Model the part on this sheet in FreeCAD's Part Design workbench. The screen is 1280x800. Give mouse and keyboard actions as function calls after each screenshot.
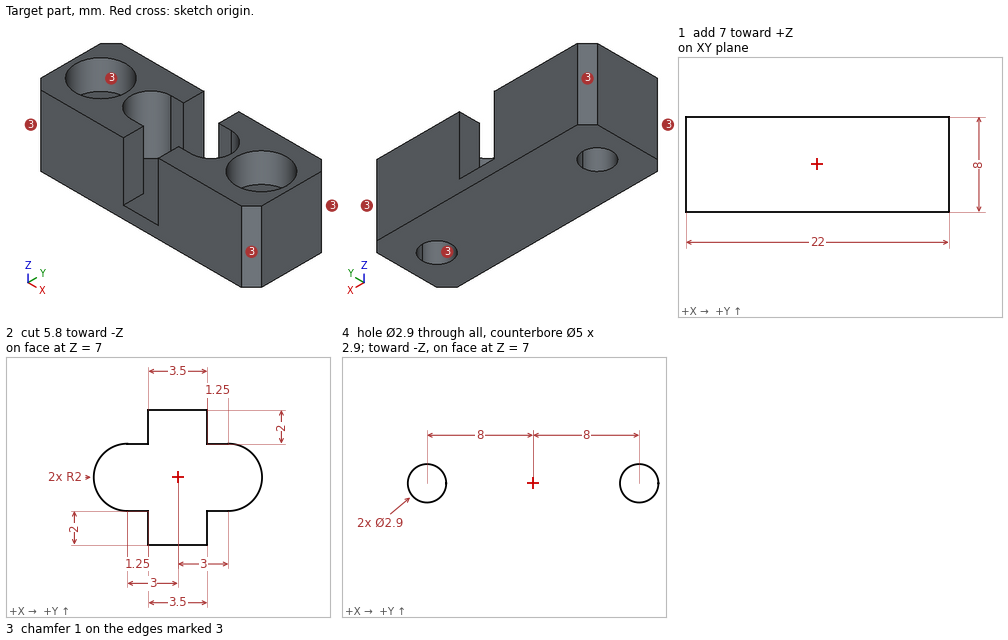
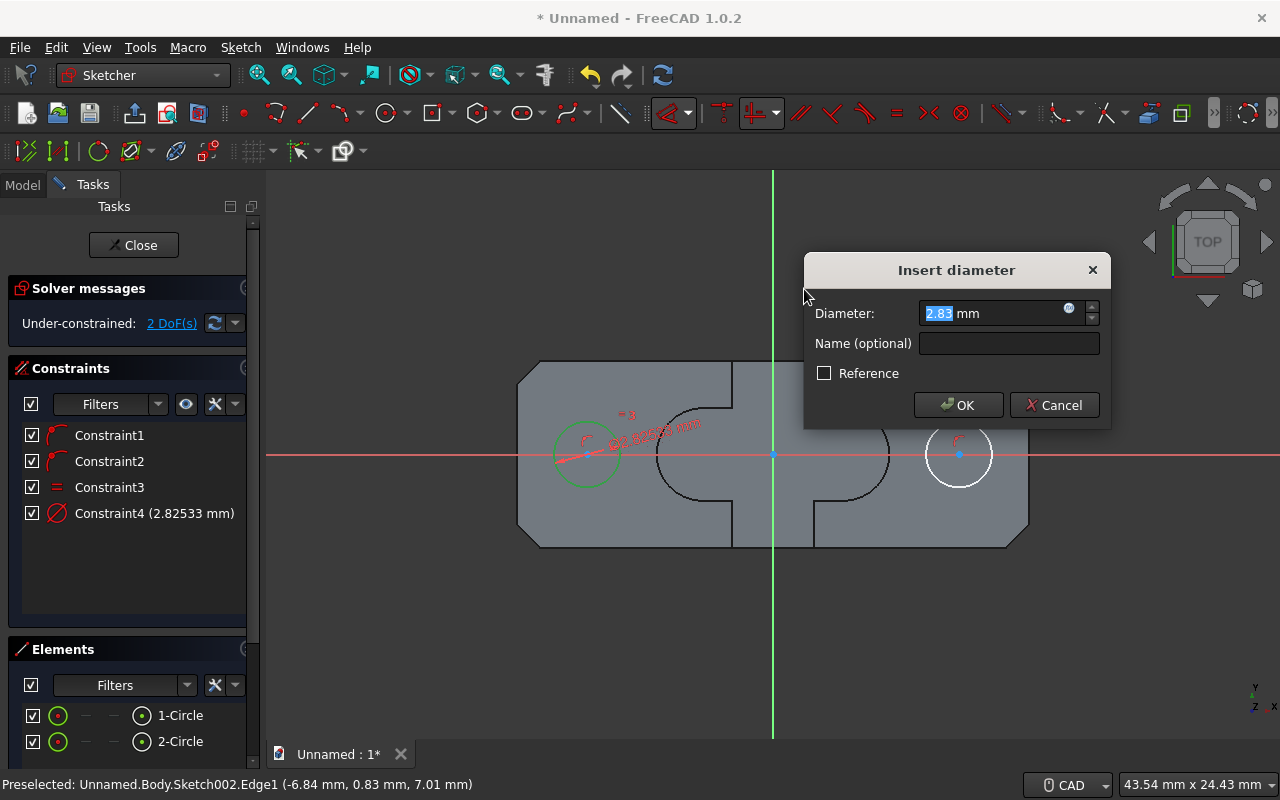
text(2.9)
key(Return)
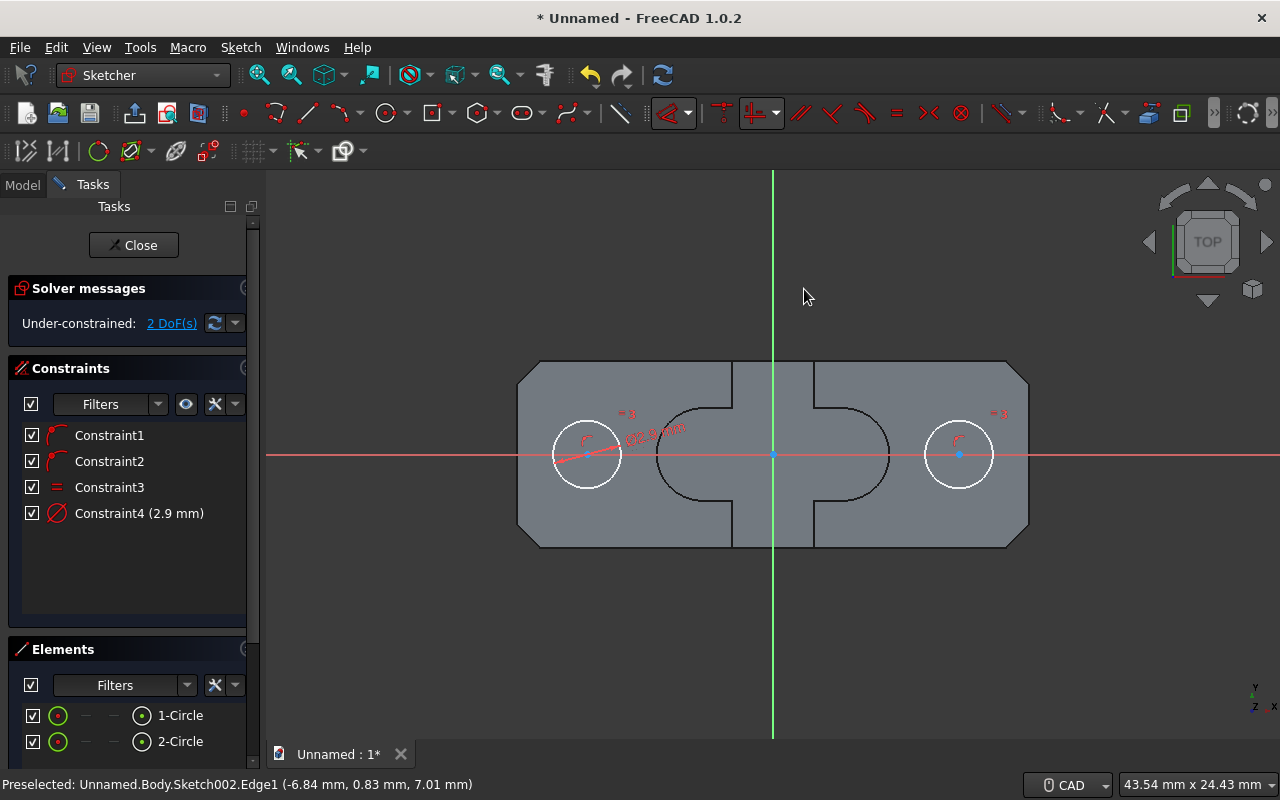
click(587, 455)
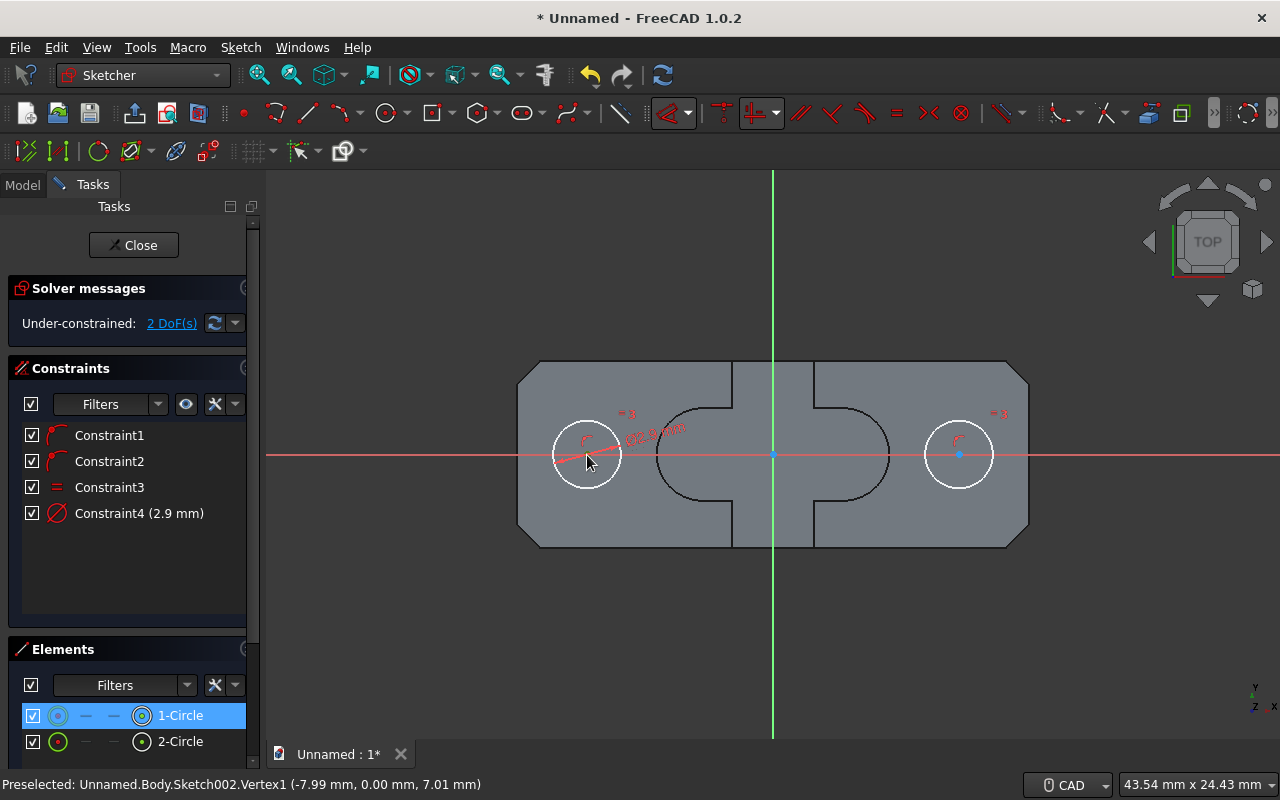
click(690, 114)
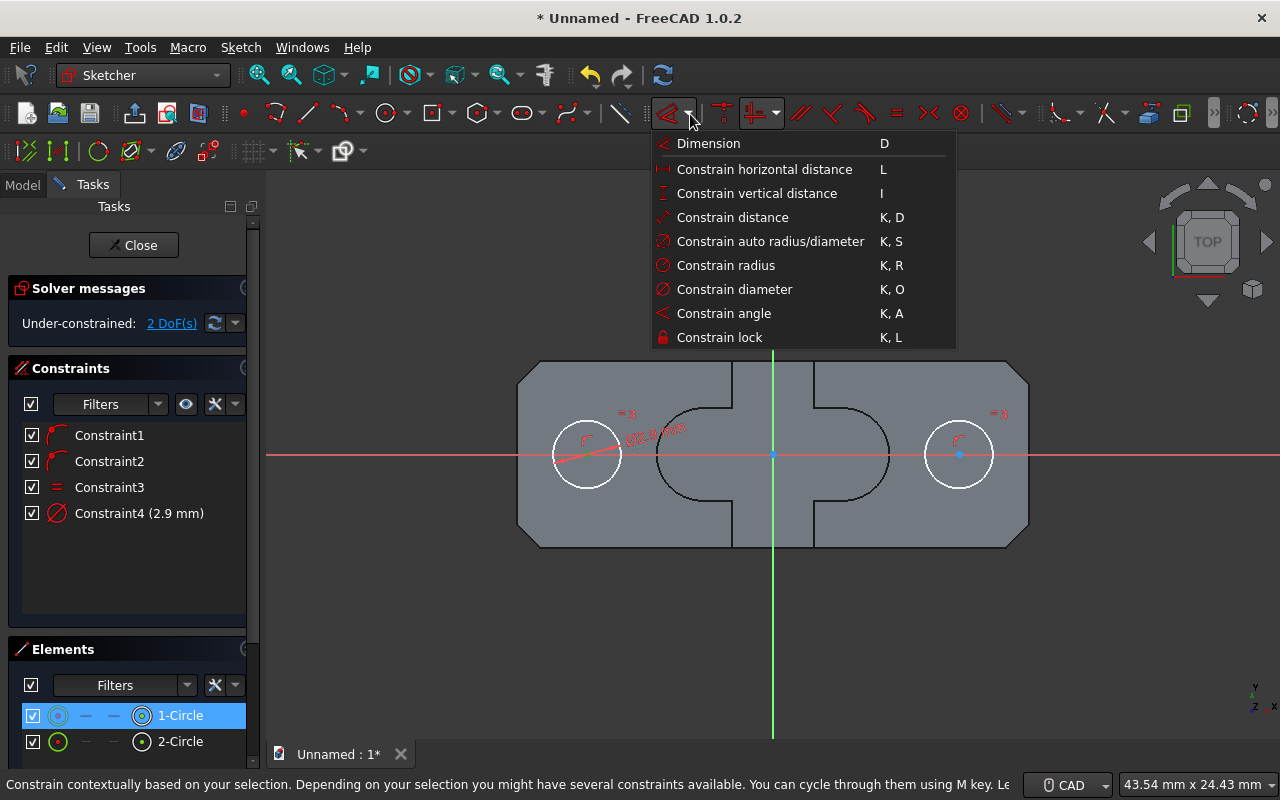
click(804, 169)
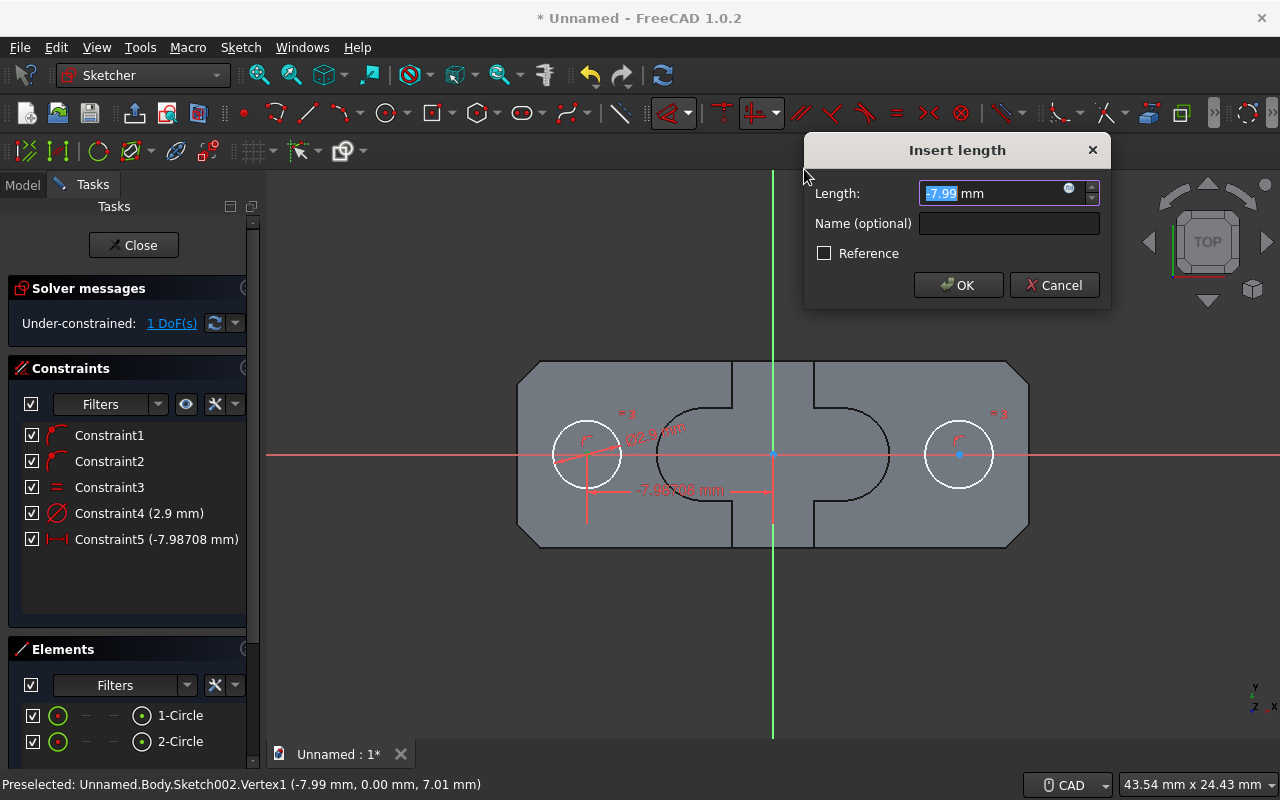
text(-8)
key(Return)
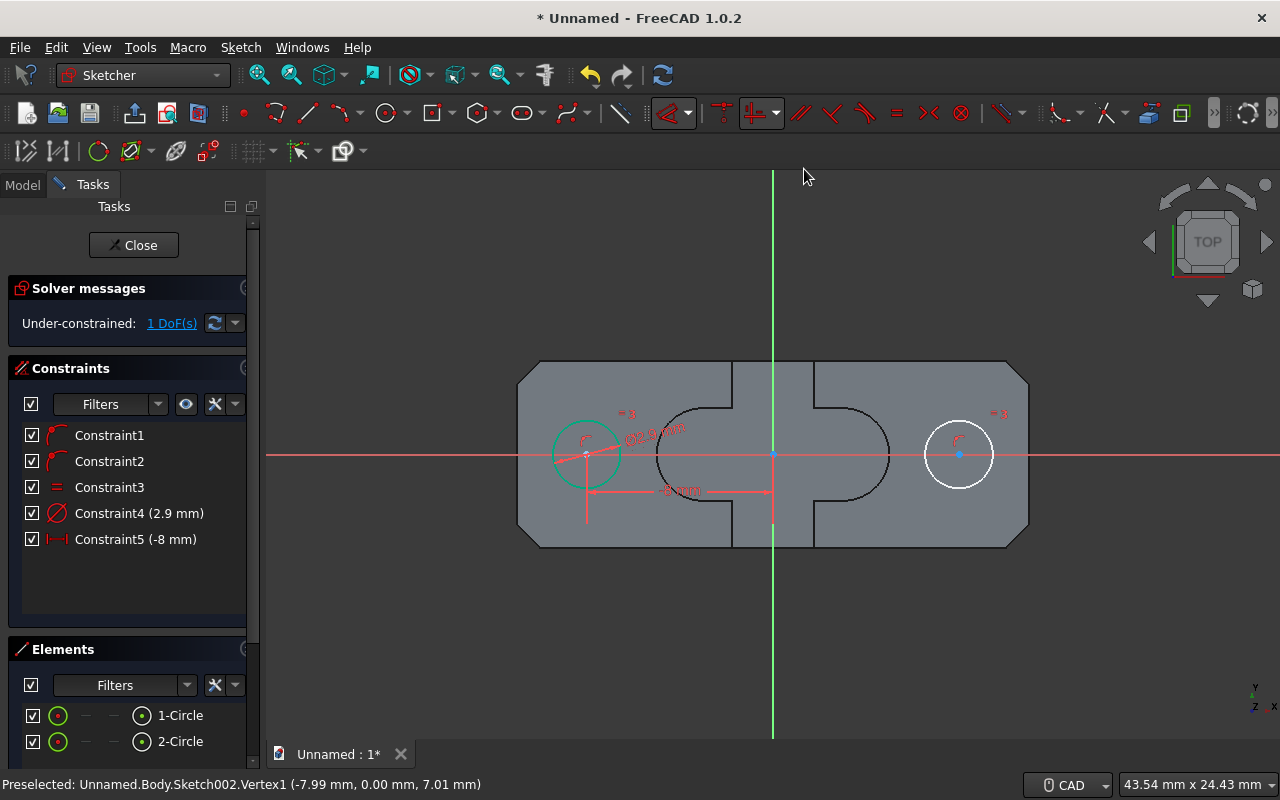
click(959, 455)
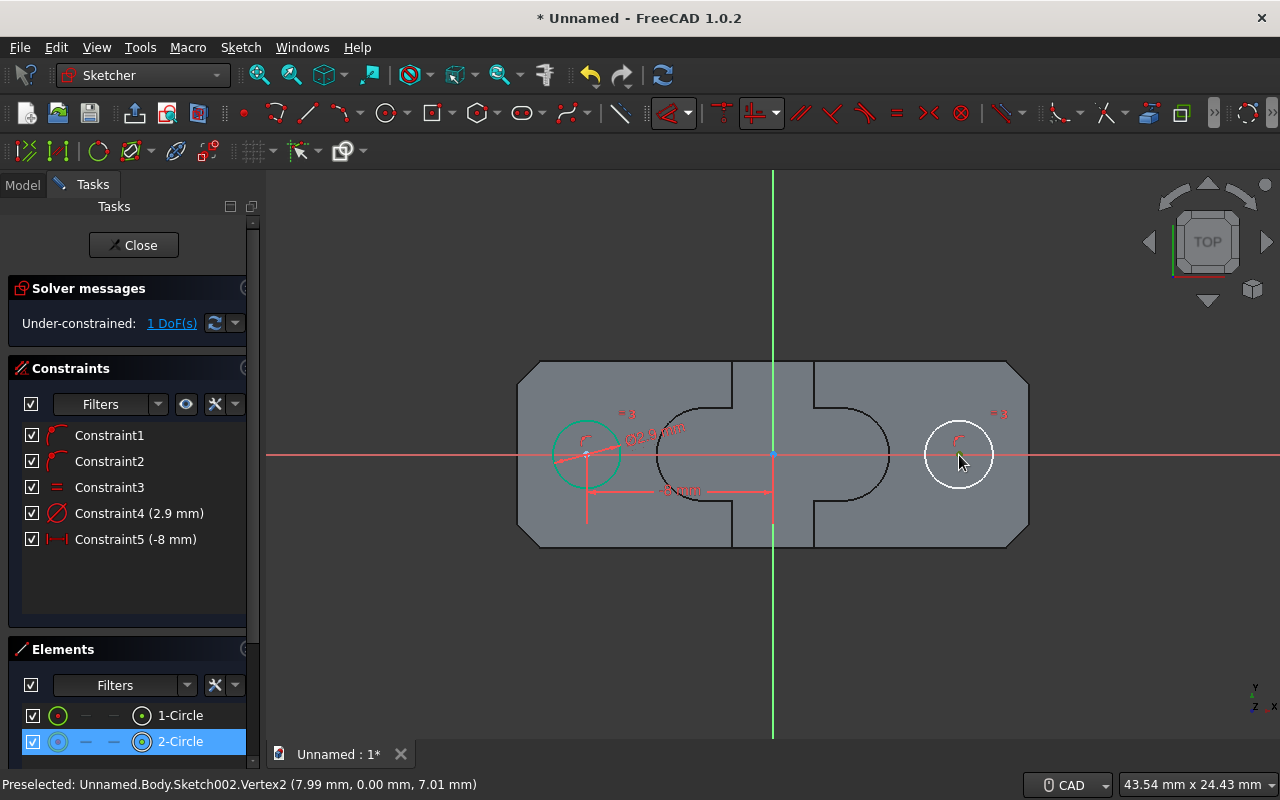
click(690, 114)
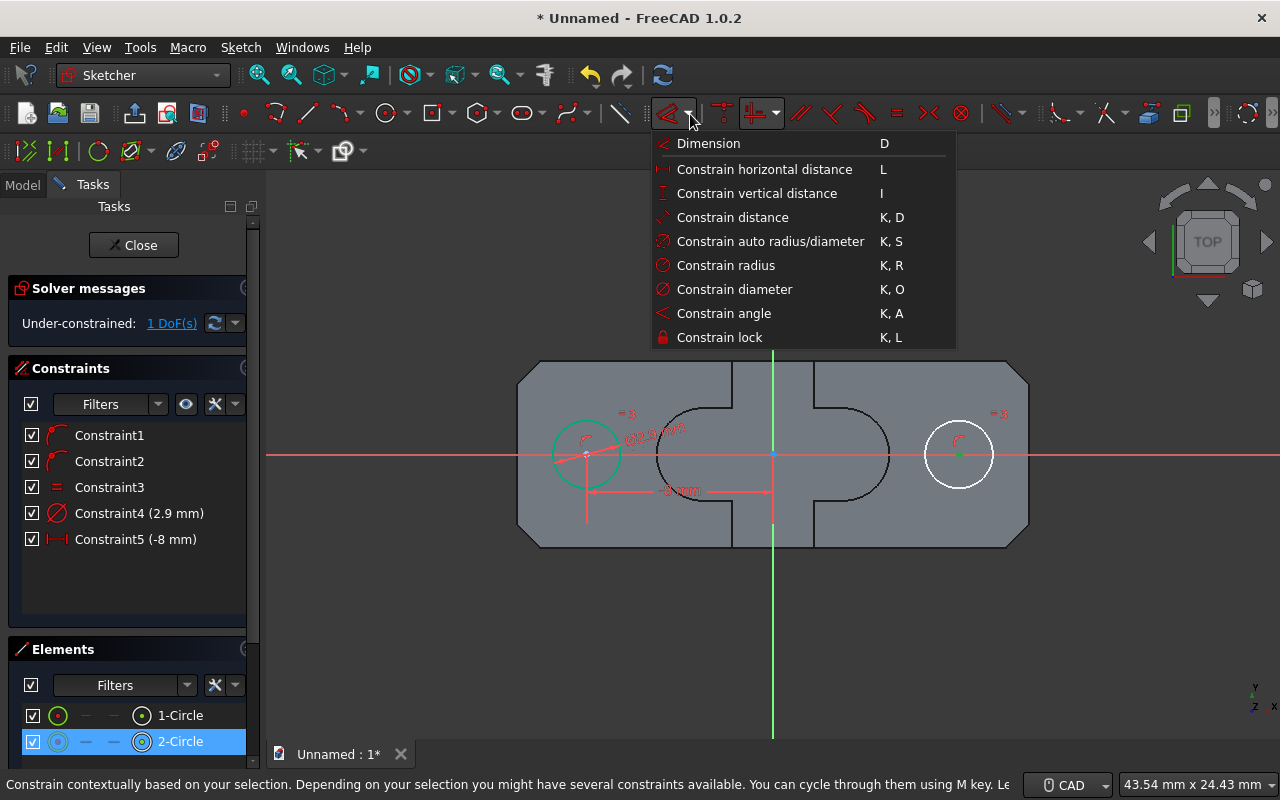
click(804, 169)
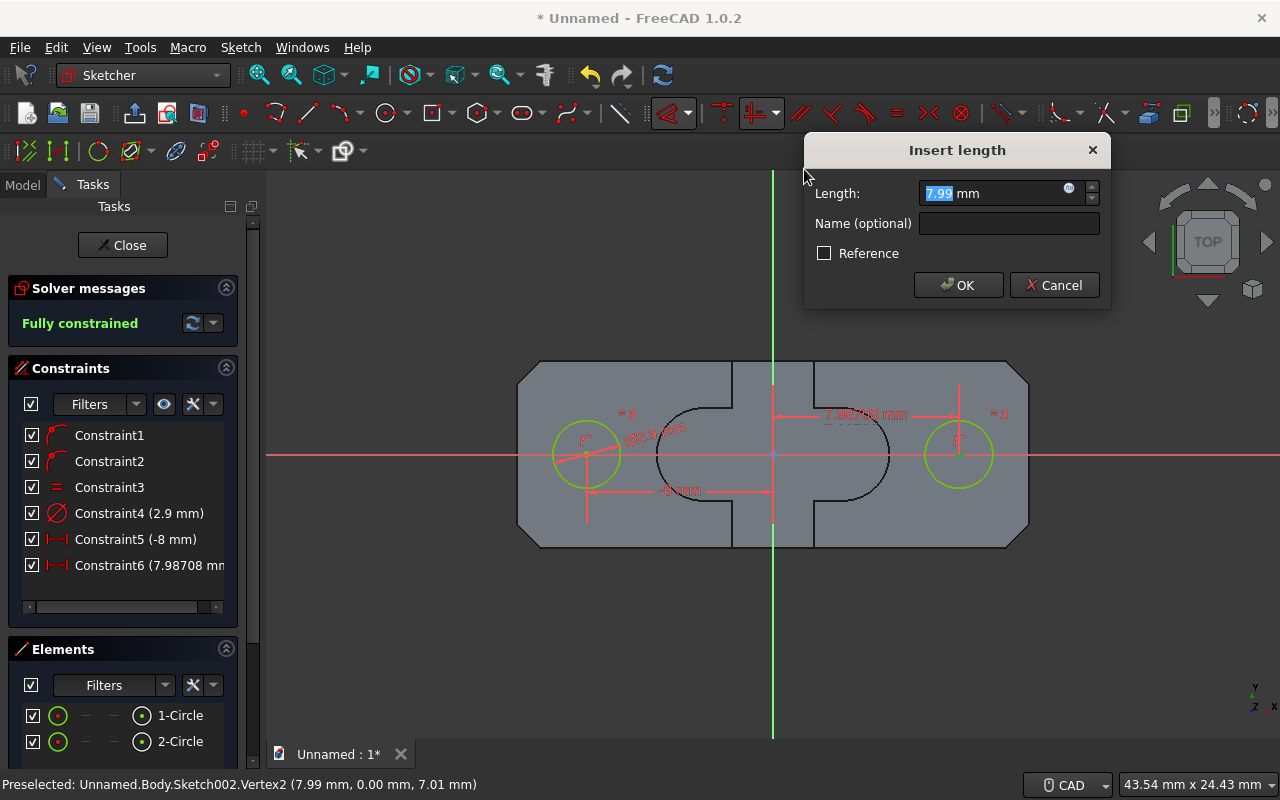
text(8)
key(Return)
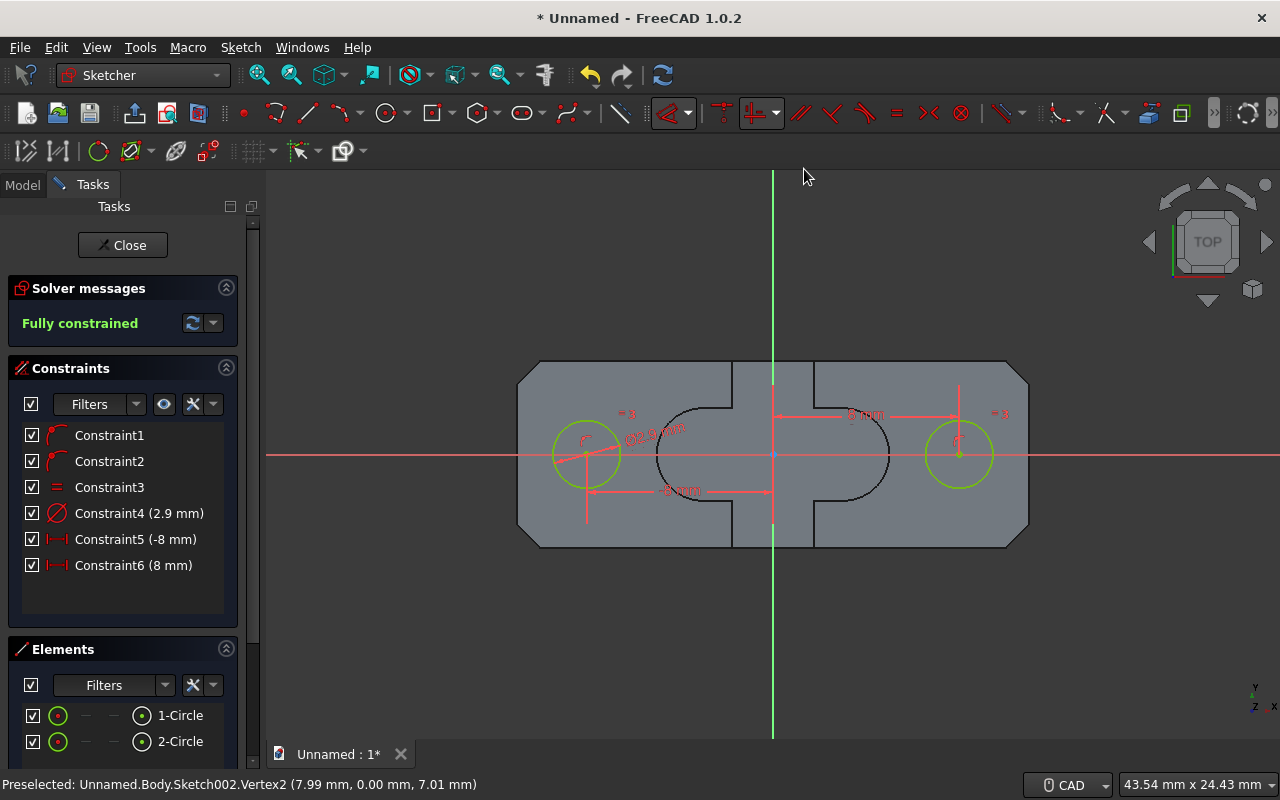
click(123, 245)